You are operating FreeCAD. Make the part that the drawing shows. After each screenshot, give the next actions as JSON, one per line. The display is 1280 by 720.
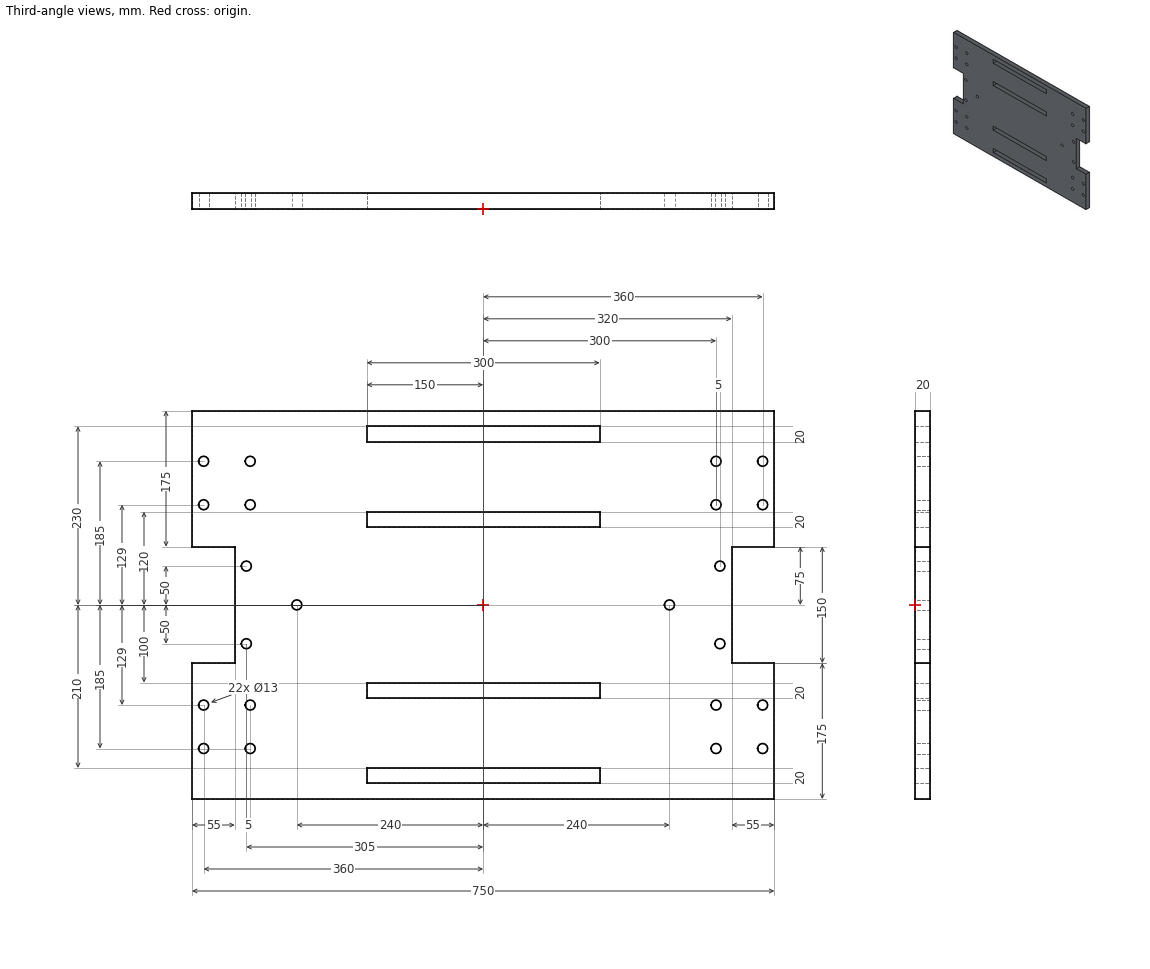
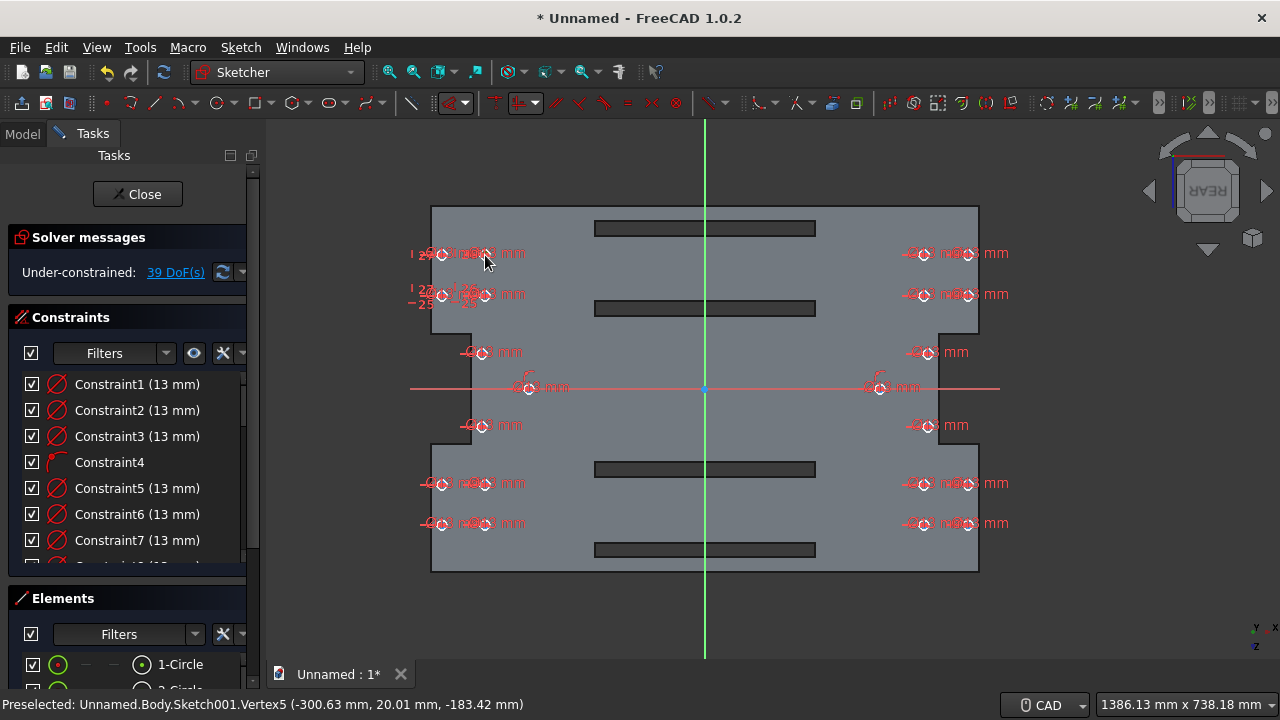
{"action": "left_click", "coordinate": [442, 255]}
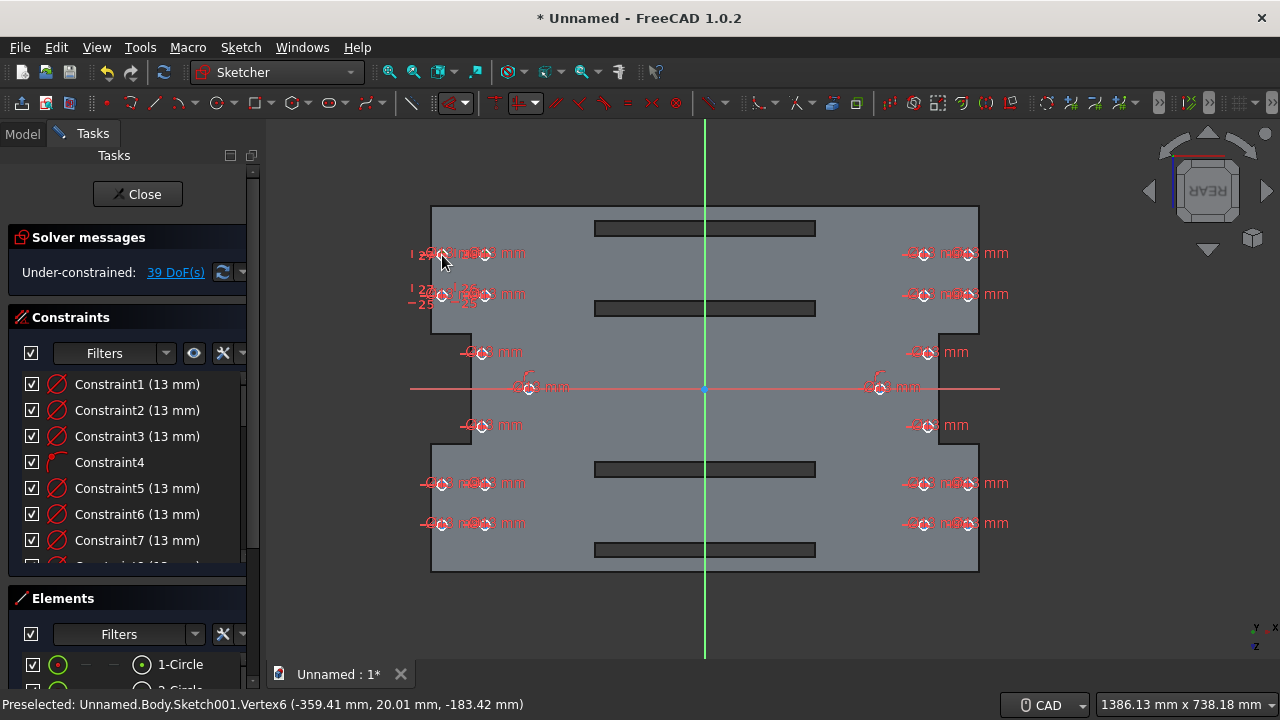
{"action": "key", "text": "h"}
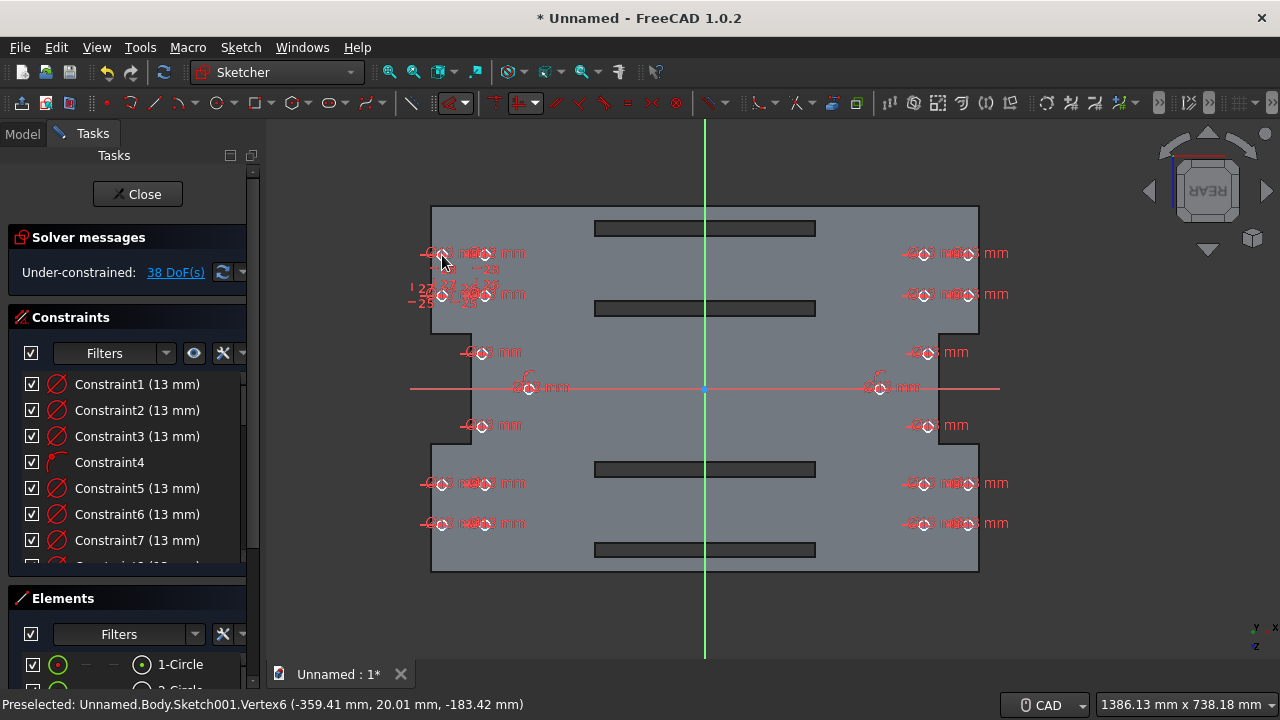
{"action": "left_click", "coordinate": [442, 296]}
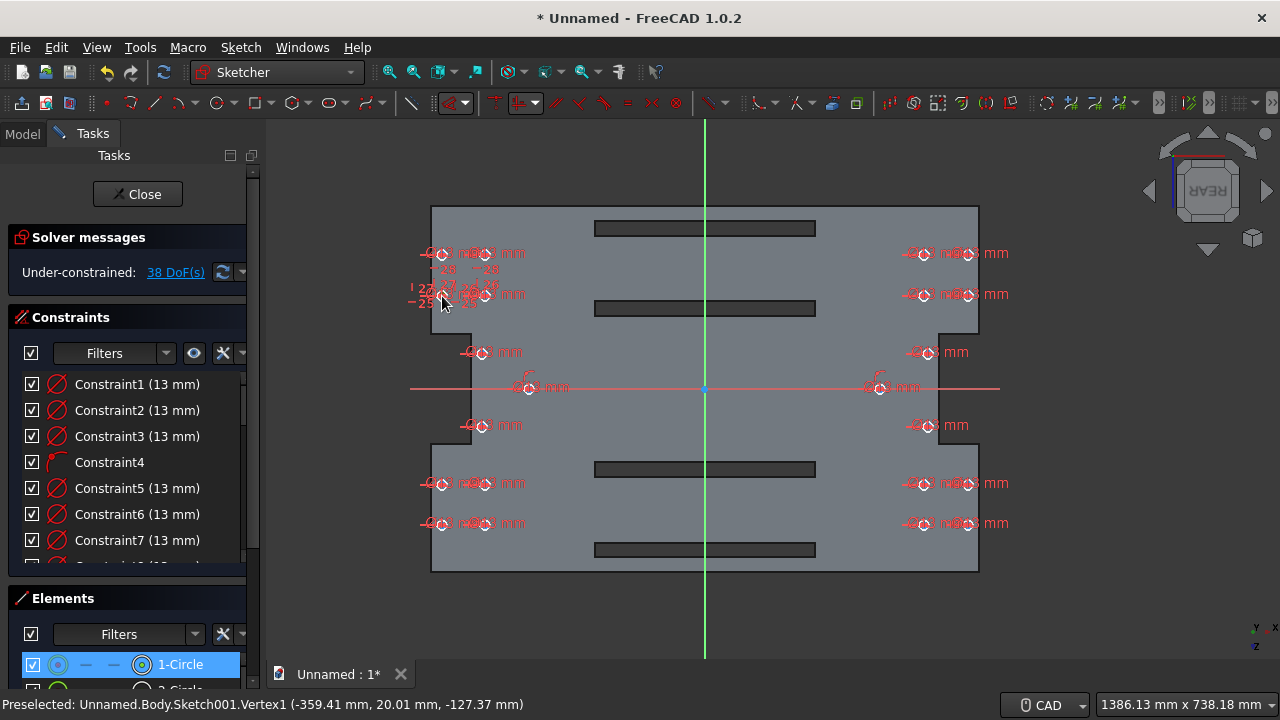
{"action": "left_click", "coordinate": [442, 485]}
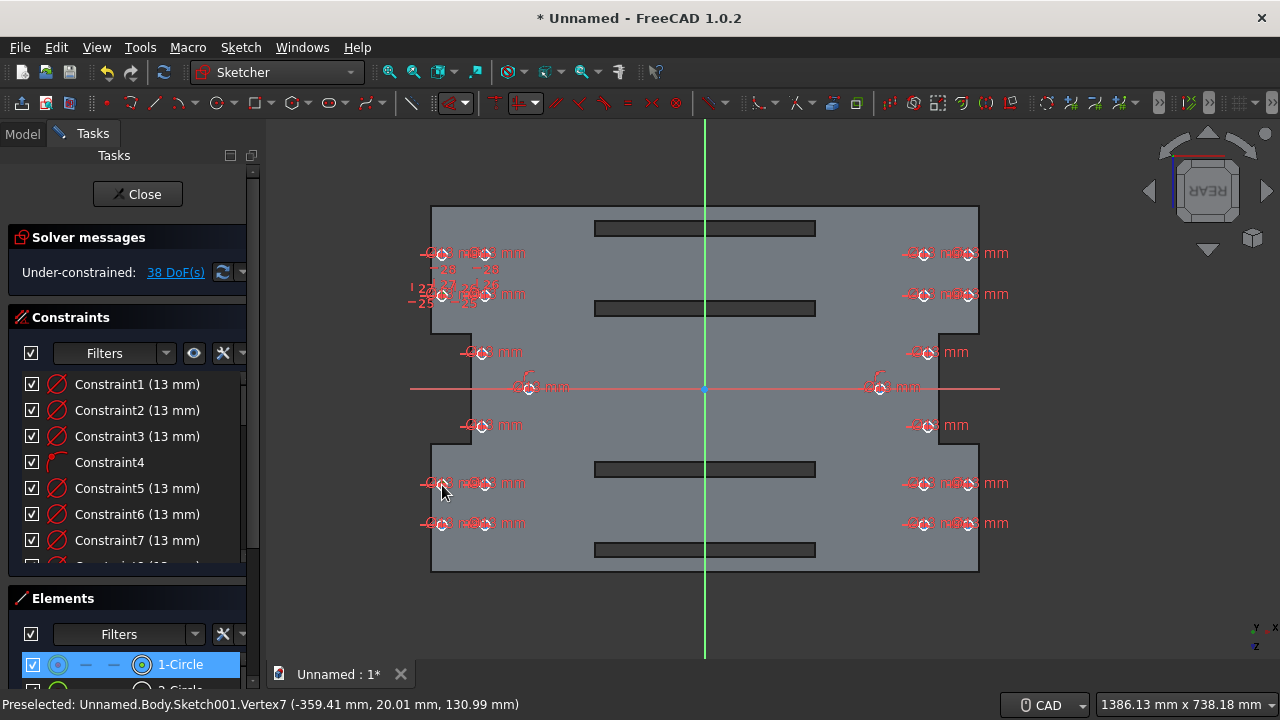
{"action": "left_click", "coordinate": [538, 104]}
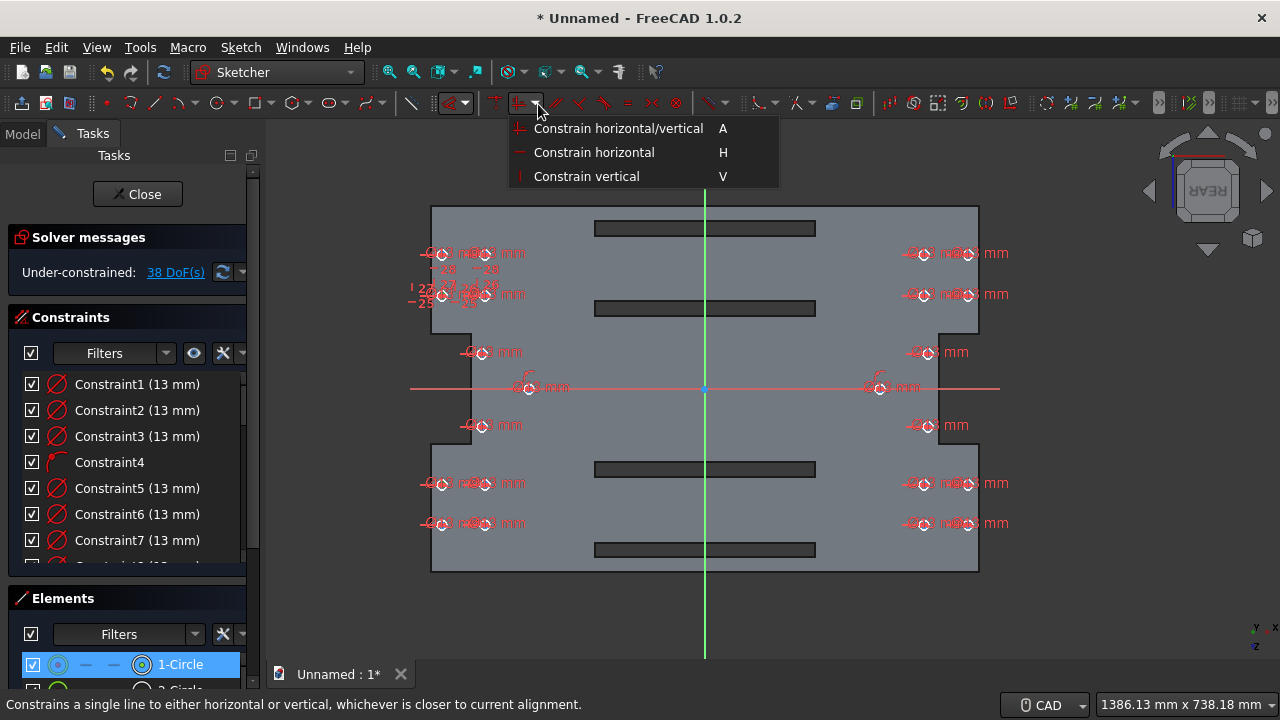
{"action": "left_click", "coordinate": [644, 176]}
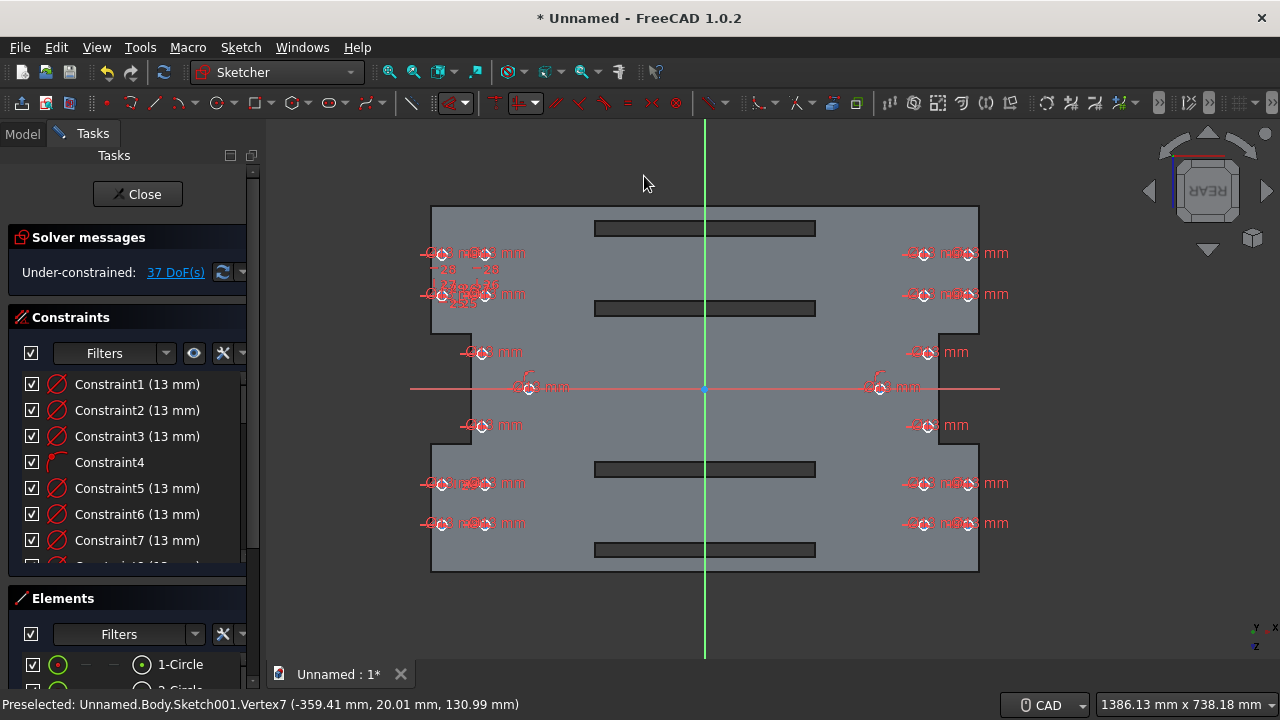
{"action": "left_click", "coordinate": [442, 485]}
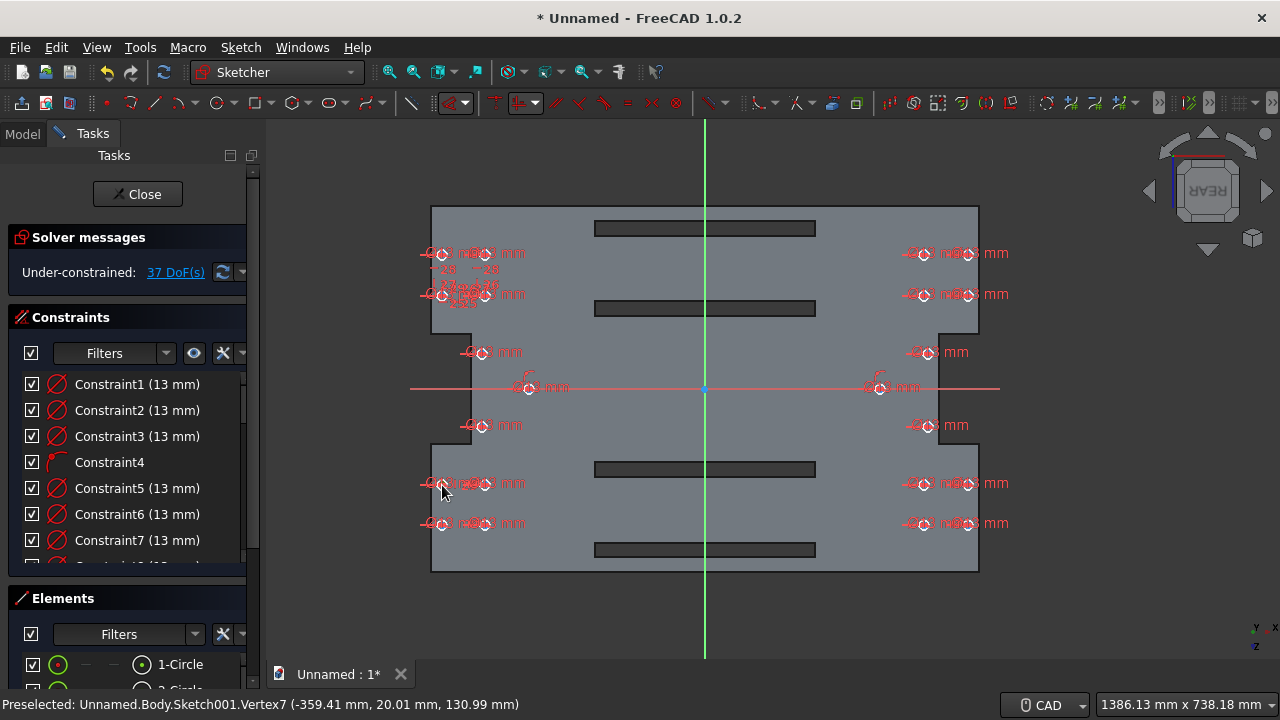
{"action": "left_click", "coordinate": [442, 525]}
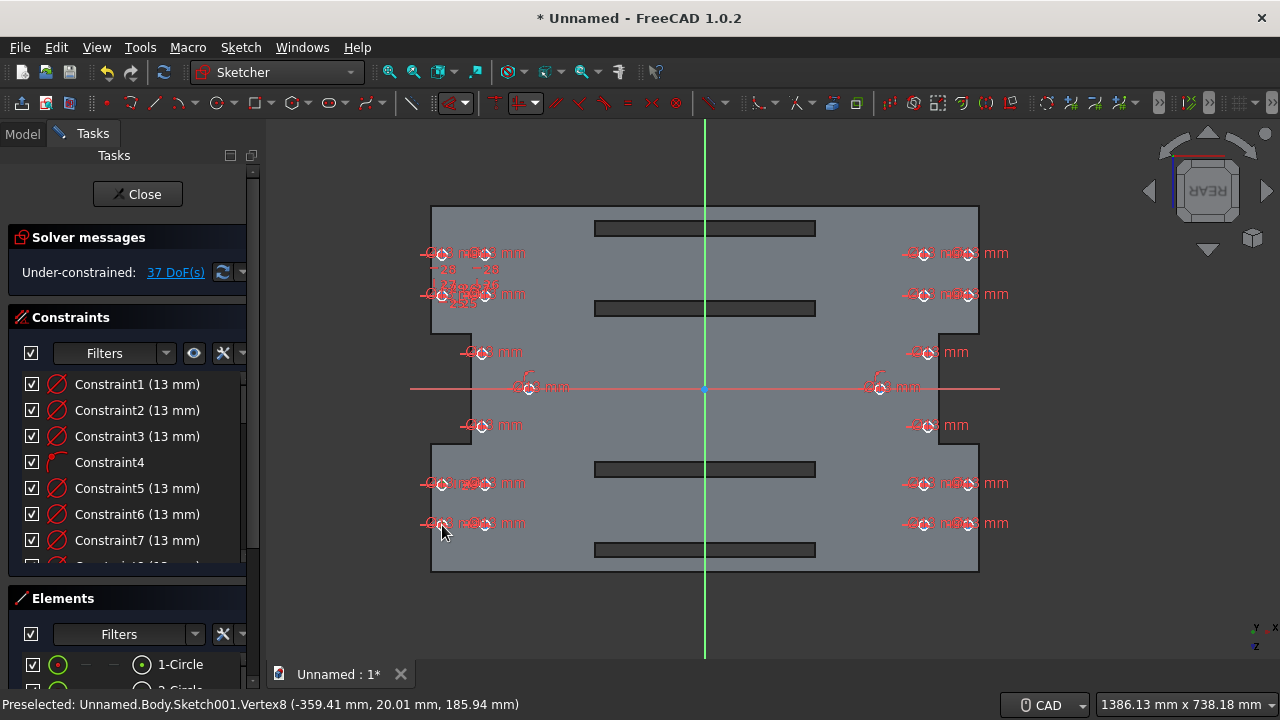
{"action": "key", "text": "v"}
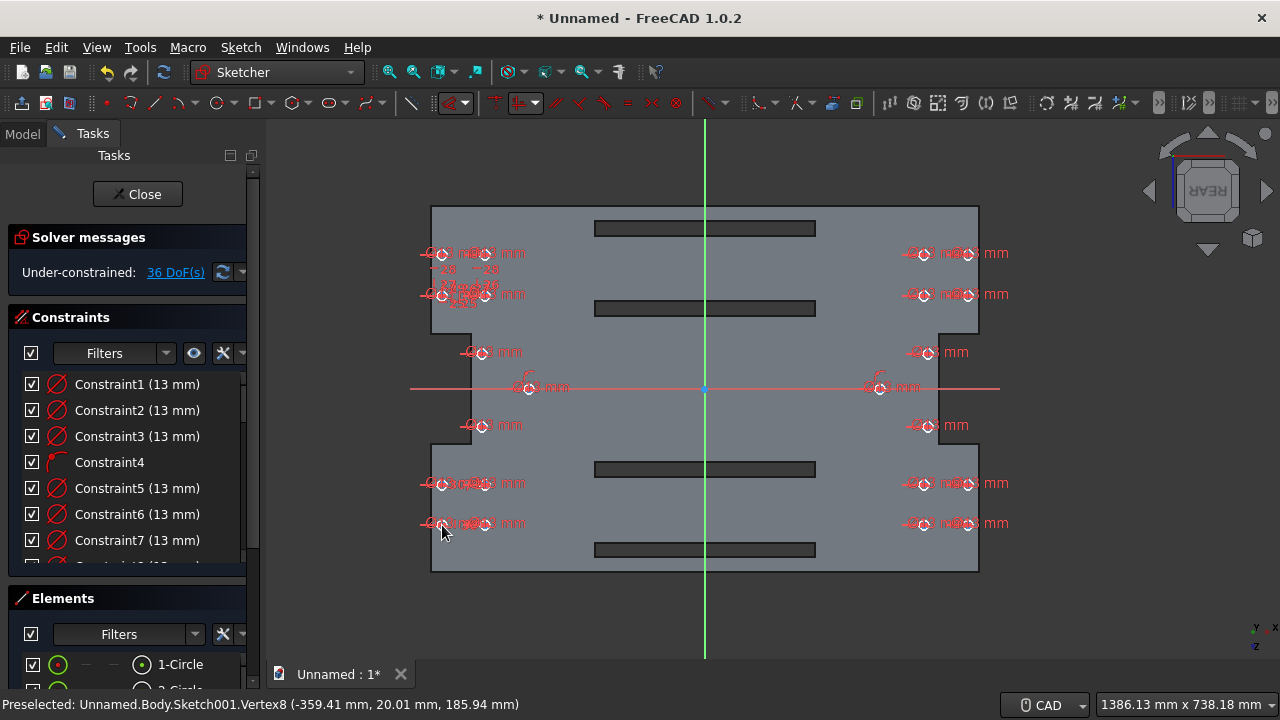
{"action": "left_click", "coordinate": [485, 296]}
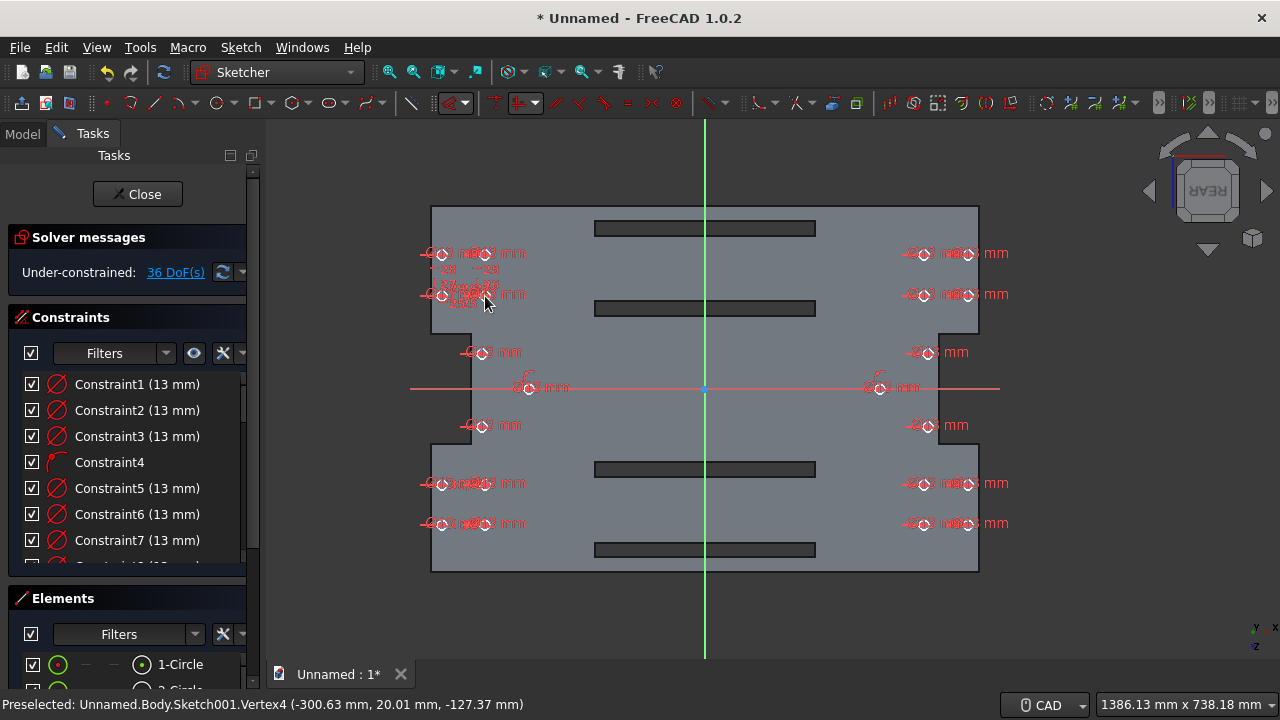
{"action": "left_click", "coordinate": [485, 485]}